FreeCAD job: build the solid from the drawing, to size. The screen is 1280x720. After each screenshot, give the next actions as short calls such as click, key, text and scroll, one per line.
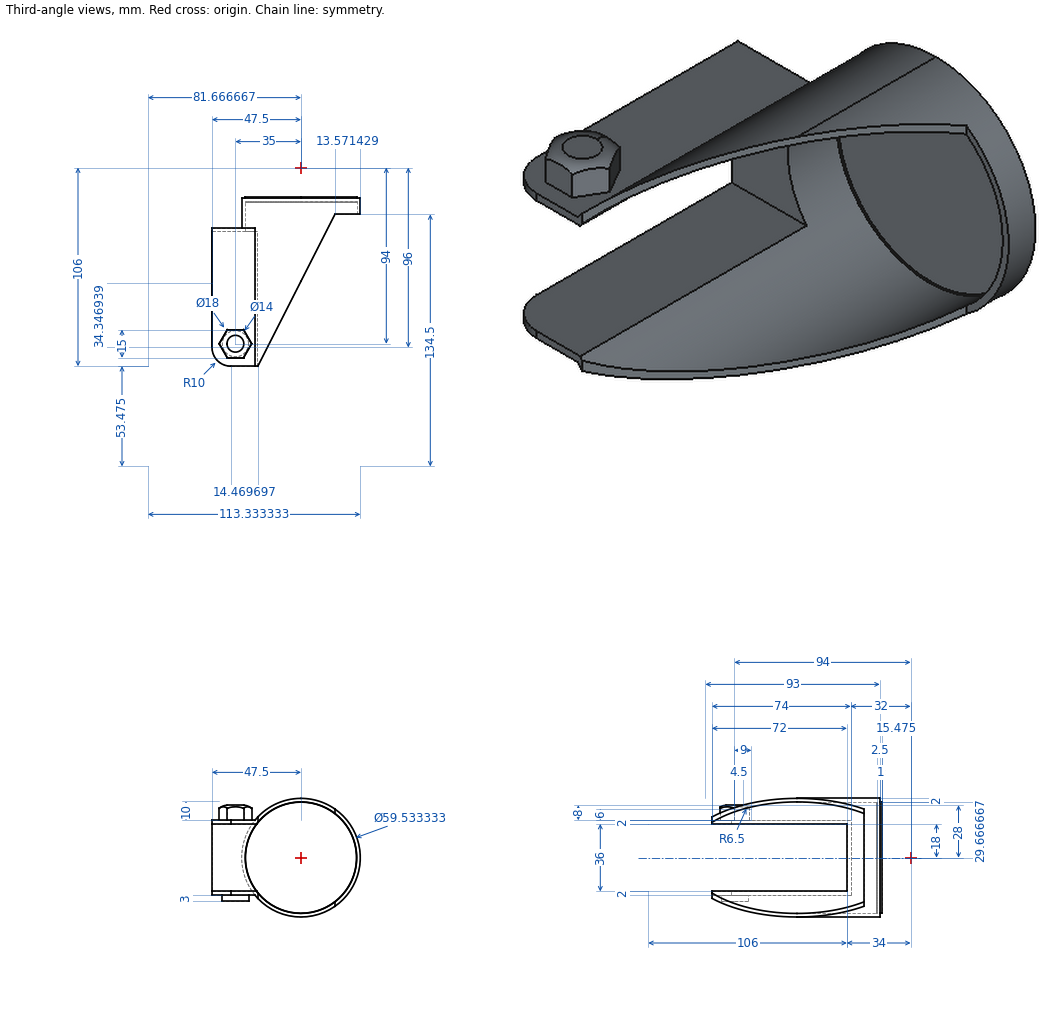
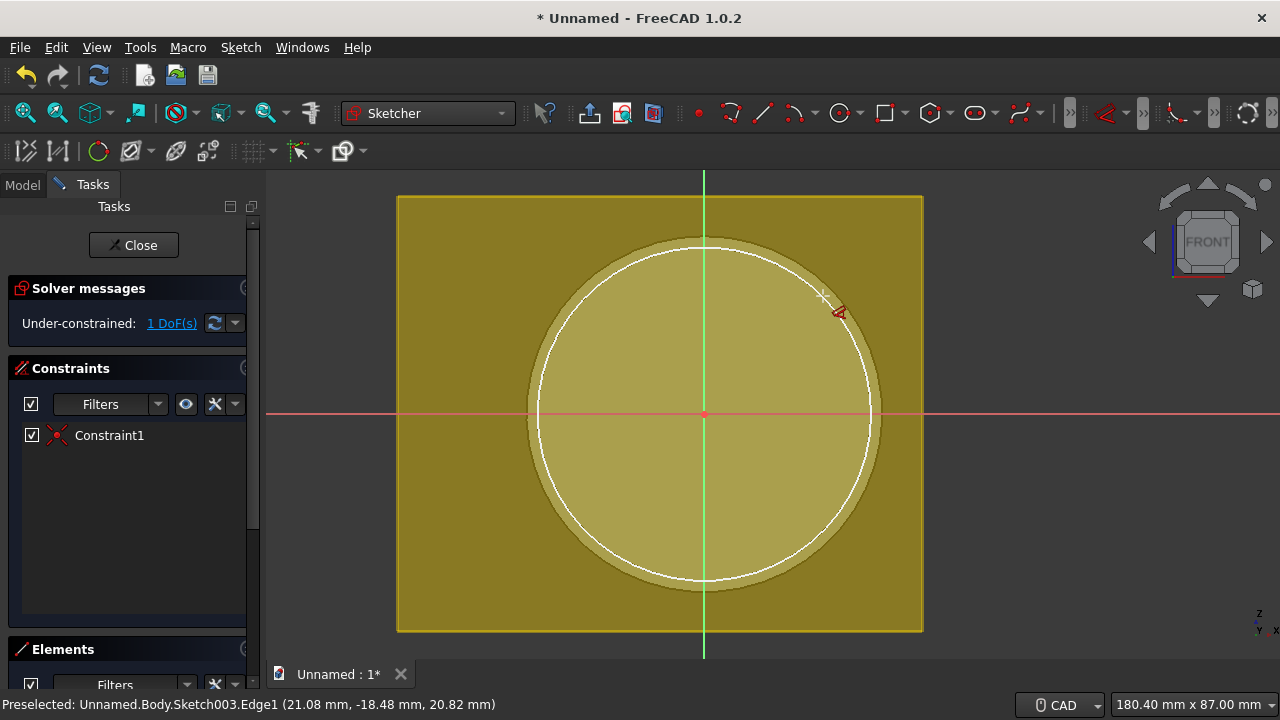
click(822, 296)
click(845, 273)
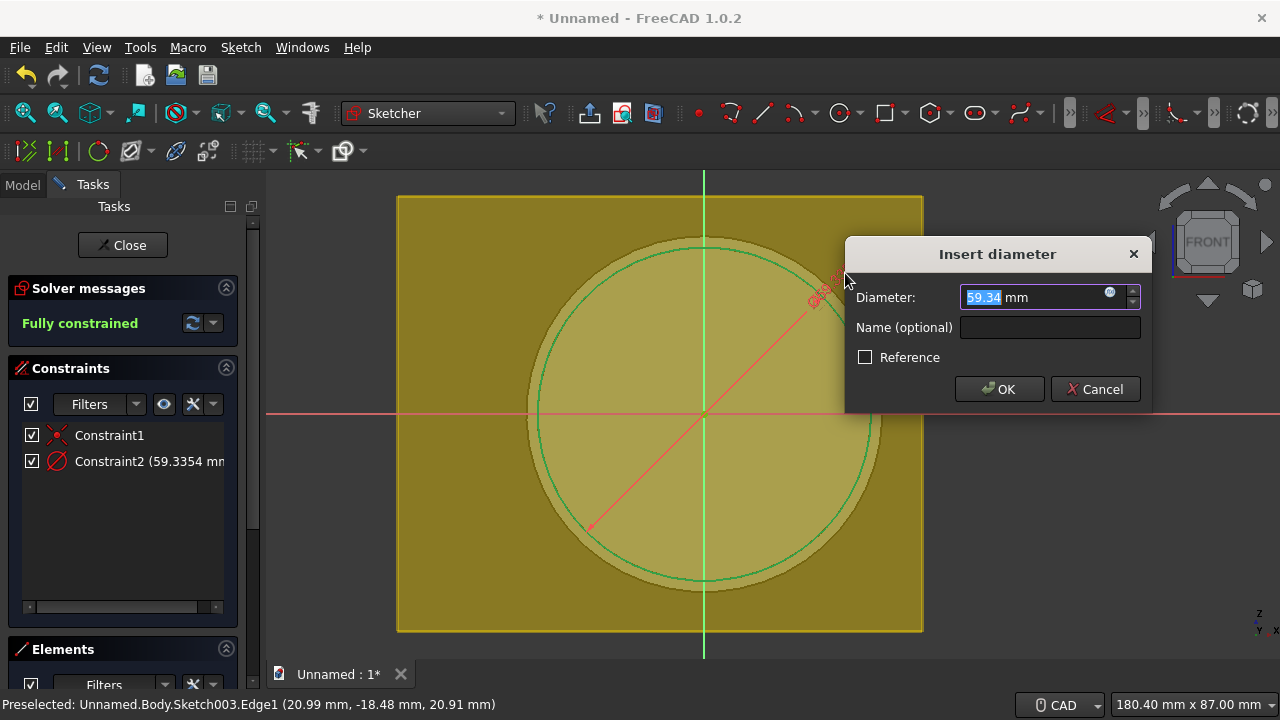
text(59.533333)
key(Return)
key(Escape)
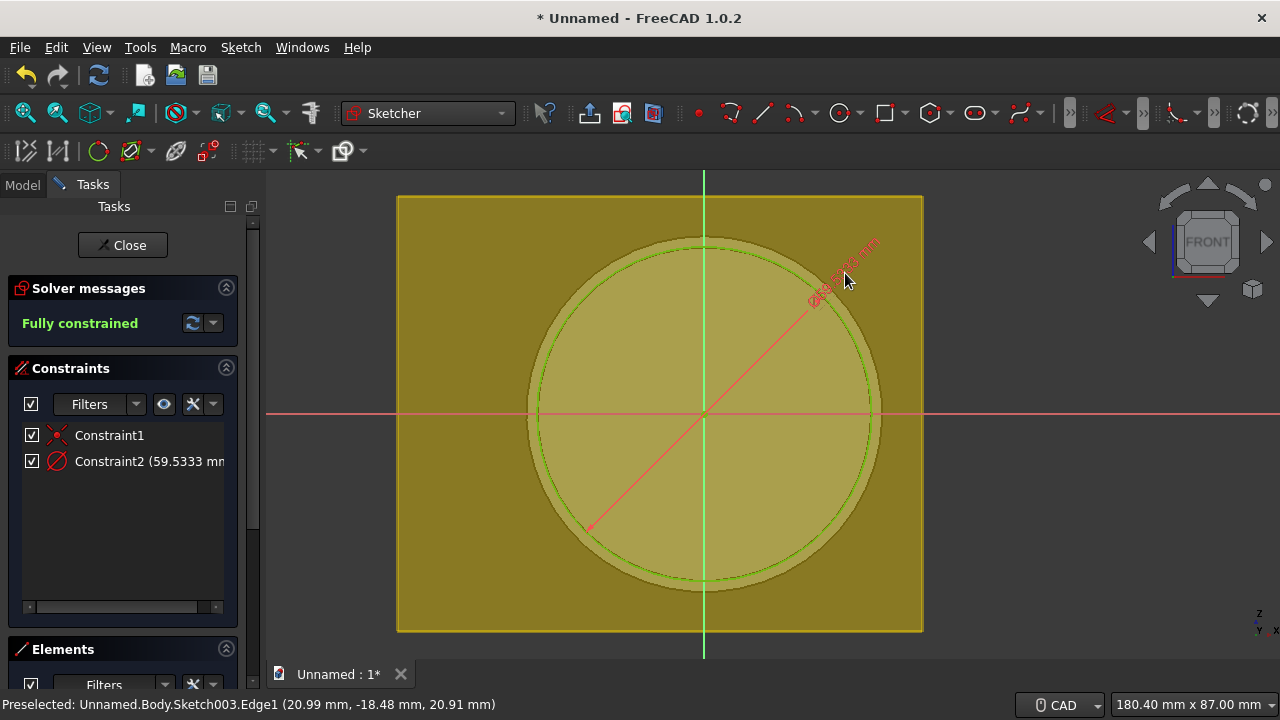
click(123, 245)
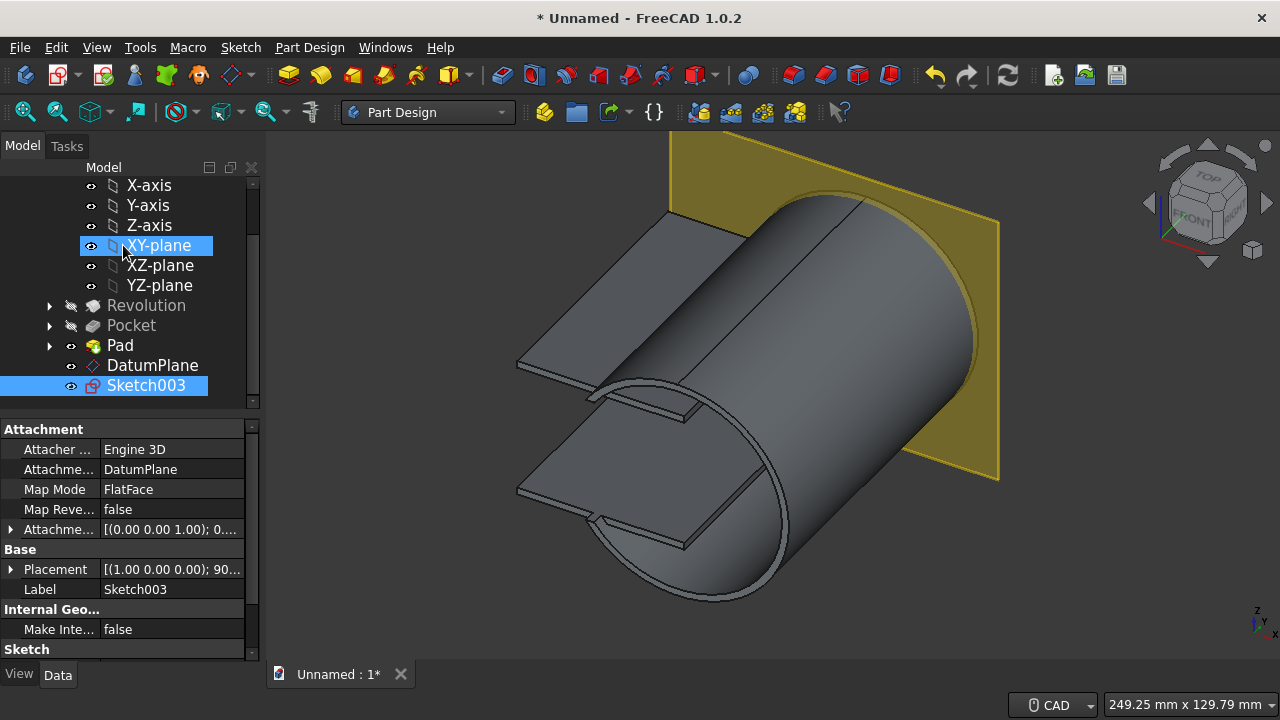
click(504, 76)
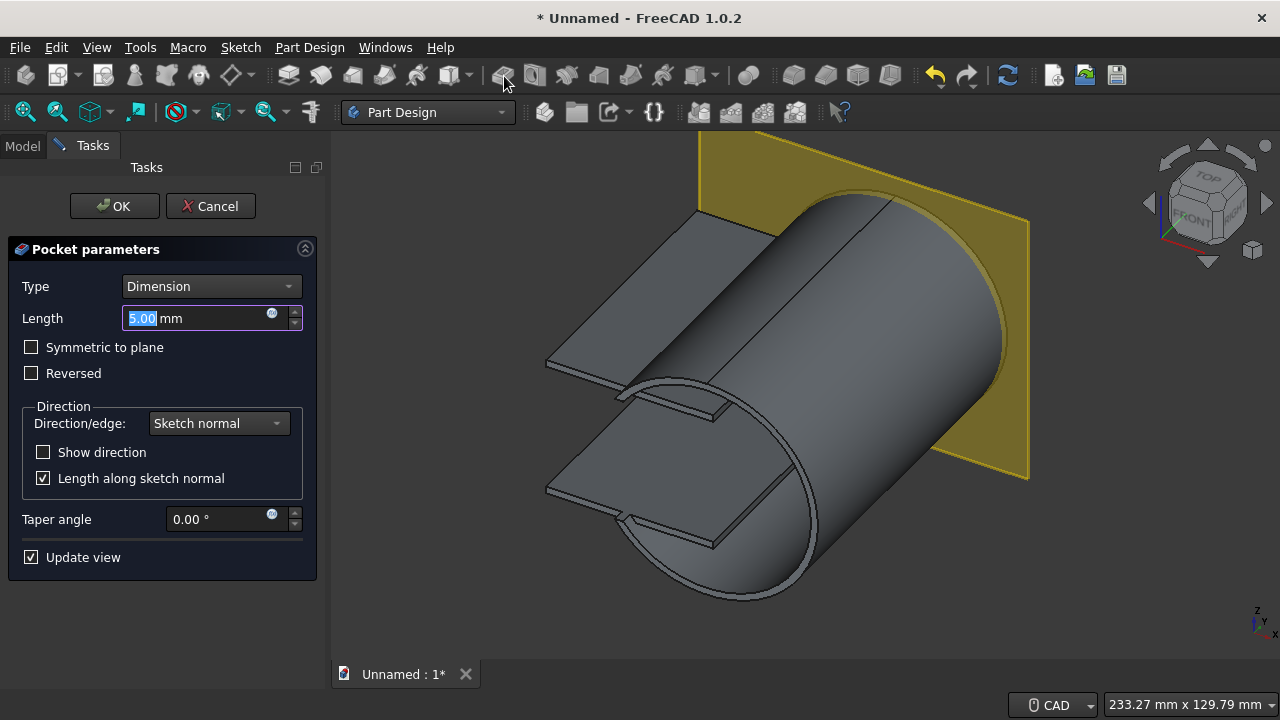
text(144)
key(Tab)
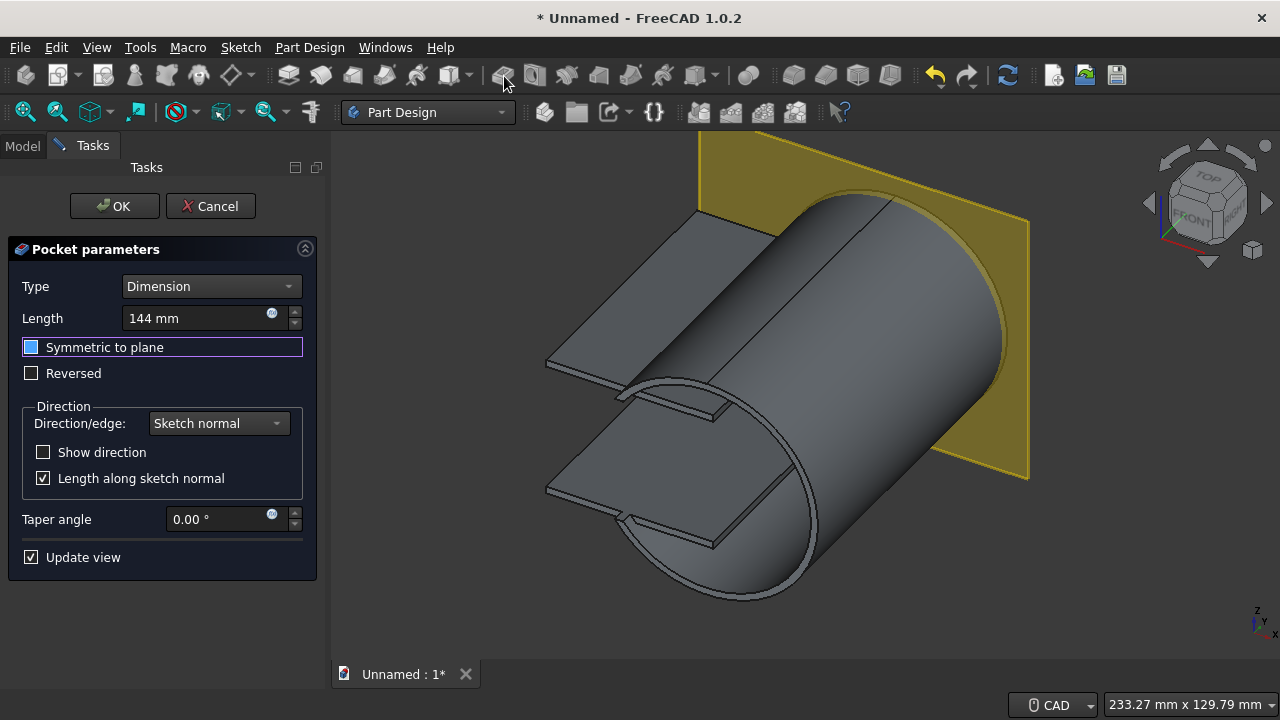
click(30, 373)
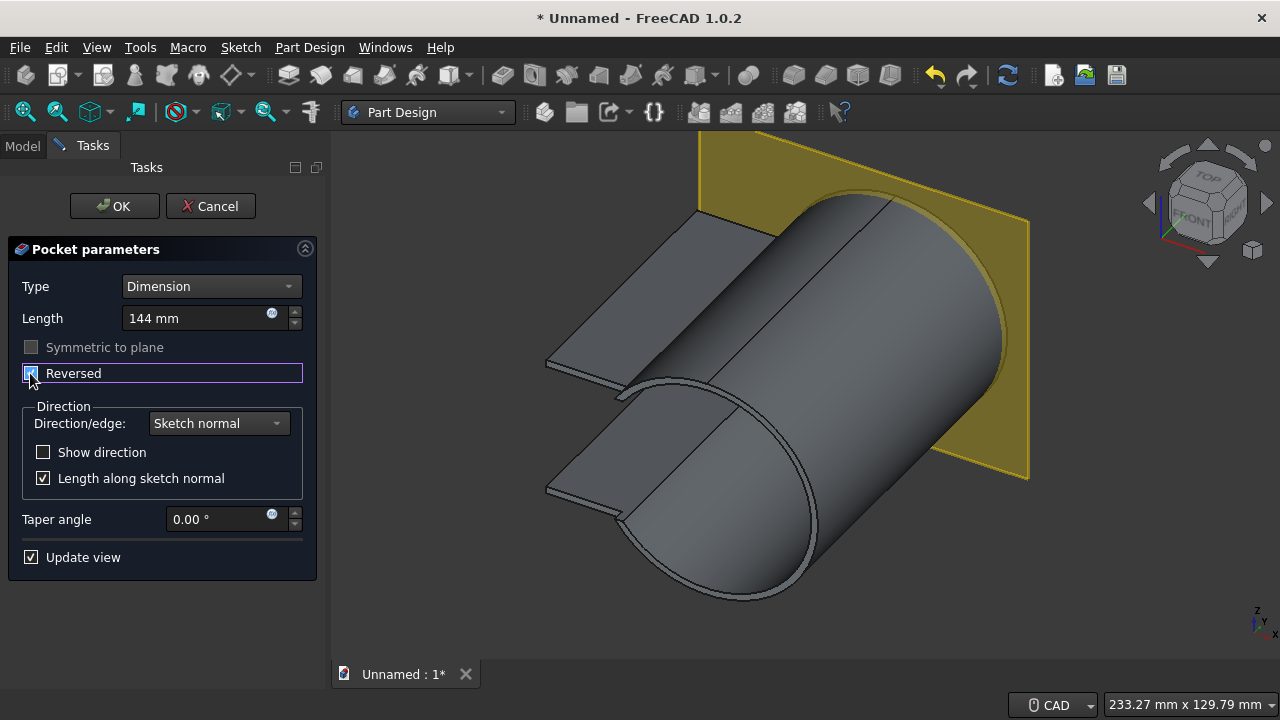
click(115, 206)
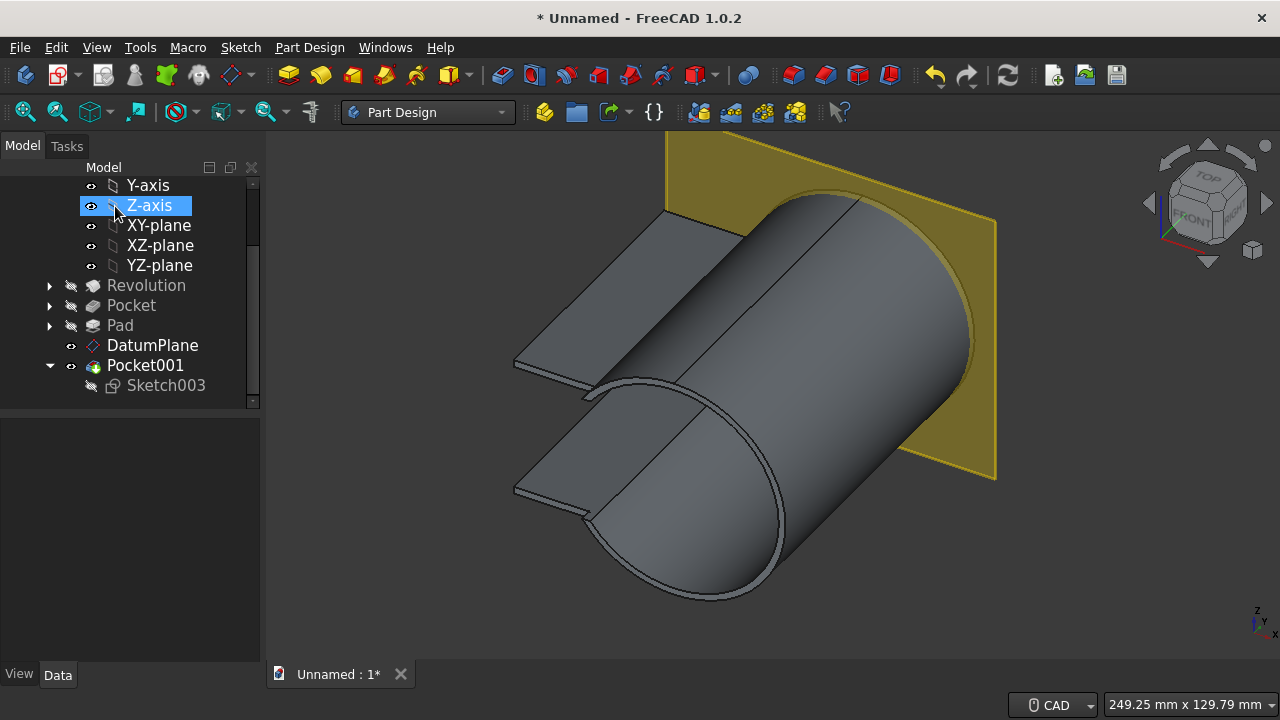
click(116, 346)
key(space)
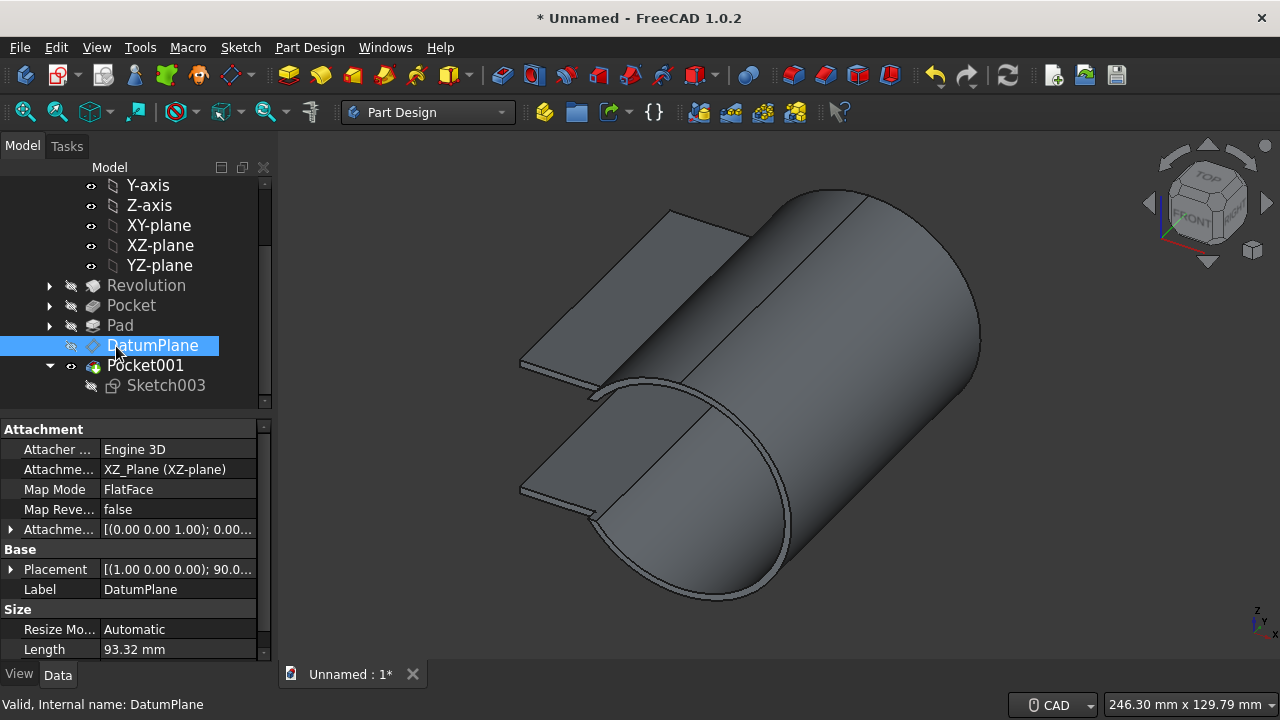
click(318, 619)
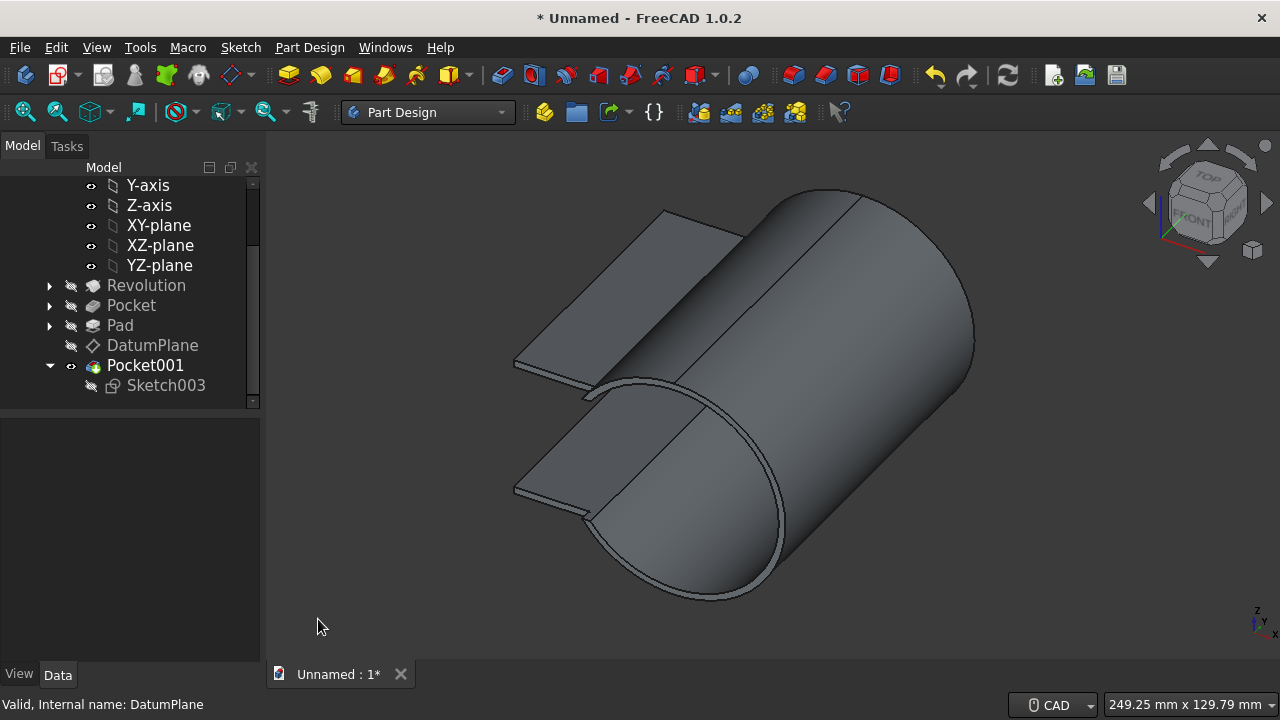
click(58, 76)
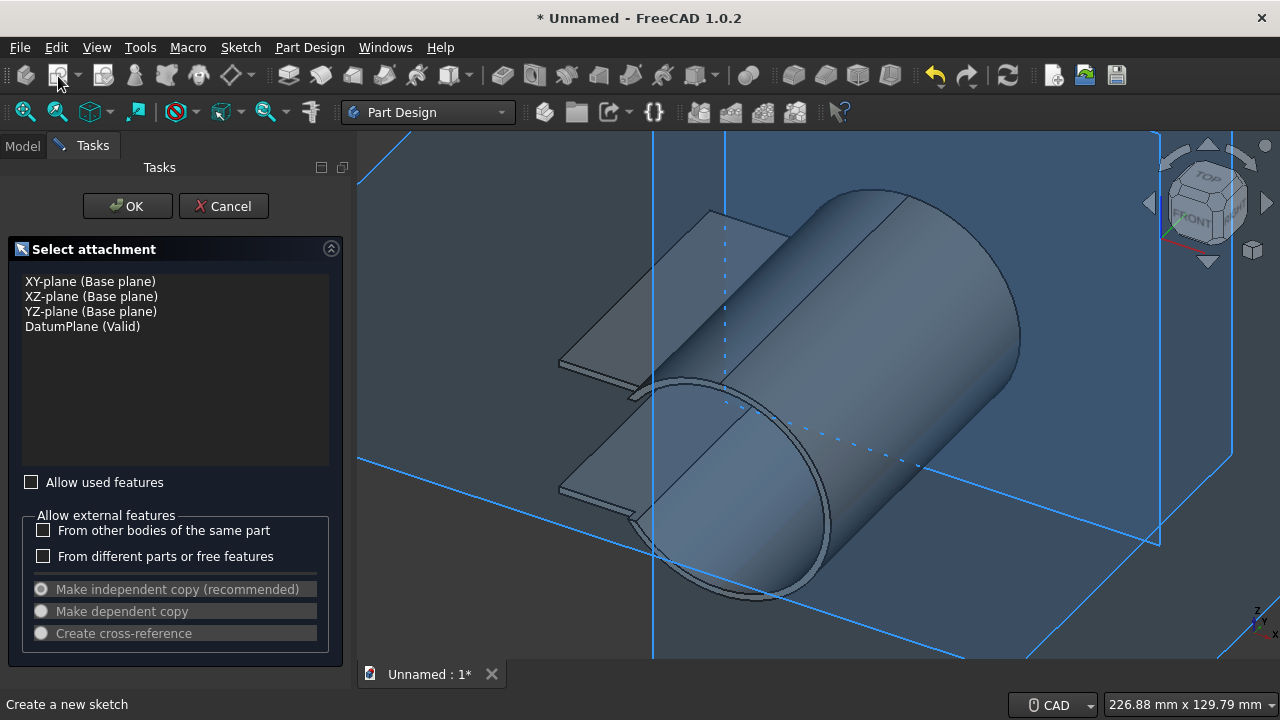
click(82, 282)